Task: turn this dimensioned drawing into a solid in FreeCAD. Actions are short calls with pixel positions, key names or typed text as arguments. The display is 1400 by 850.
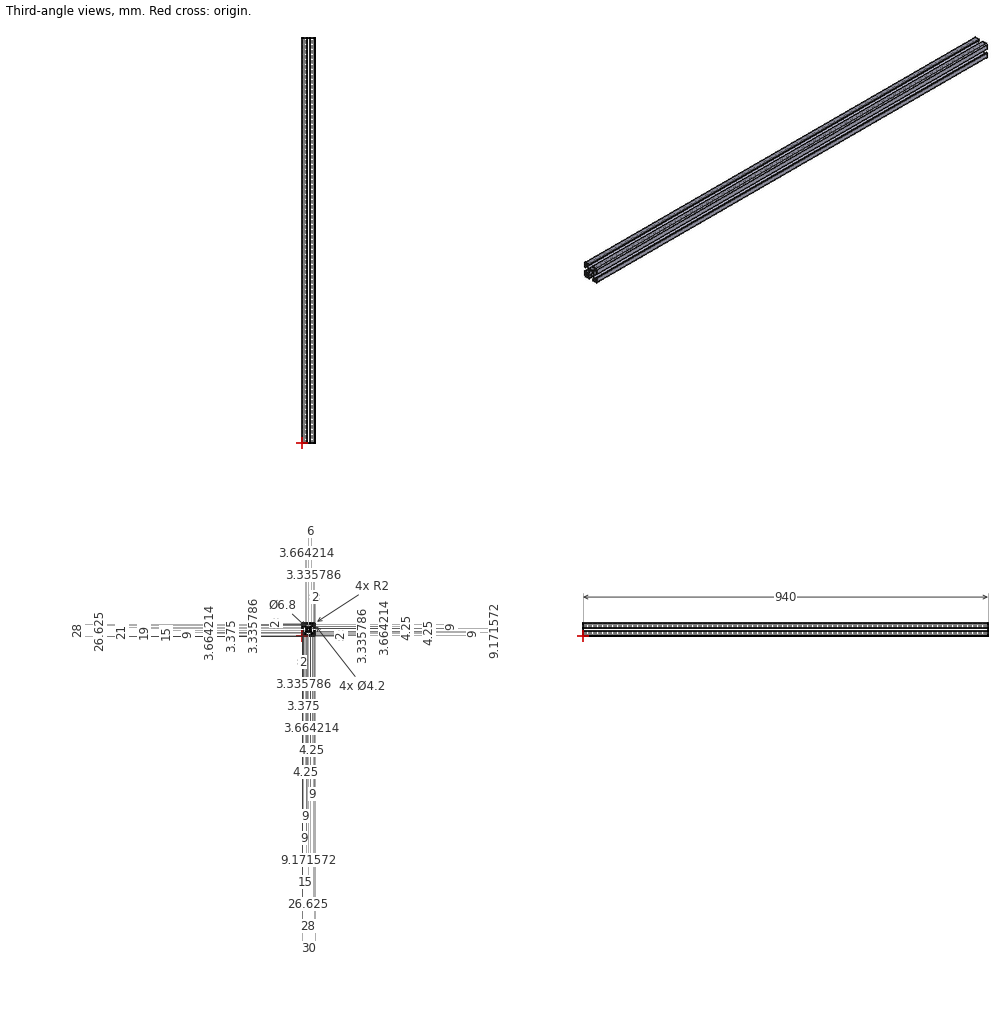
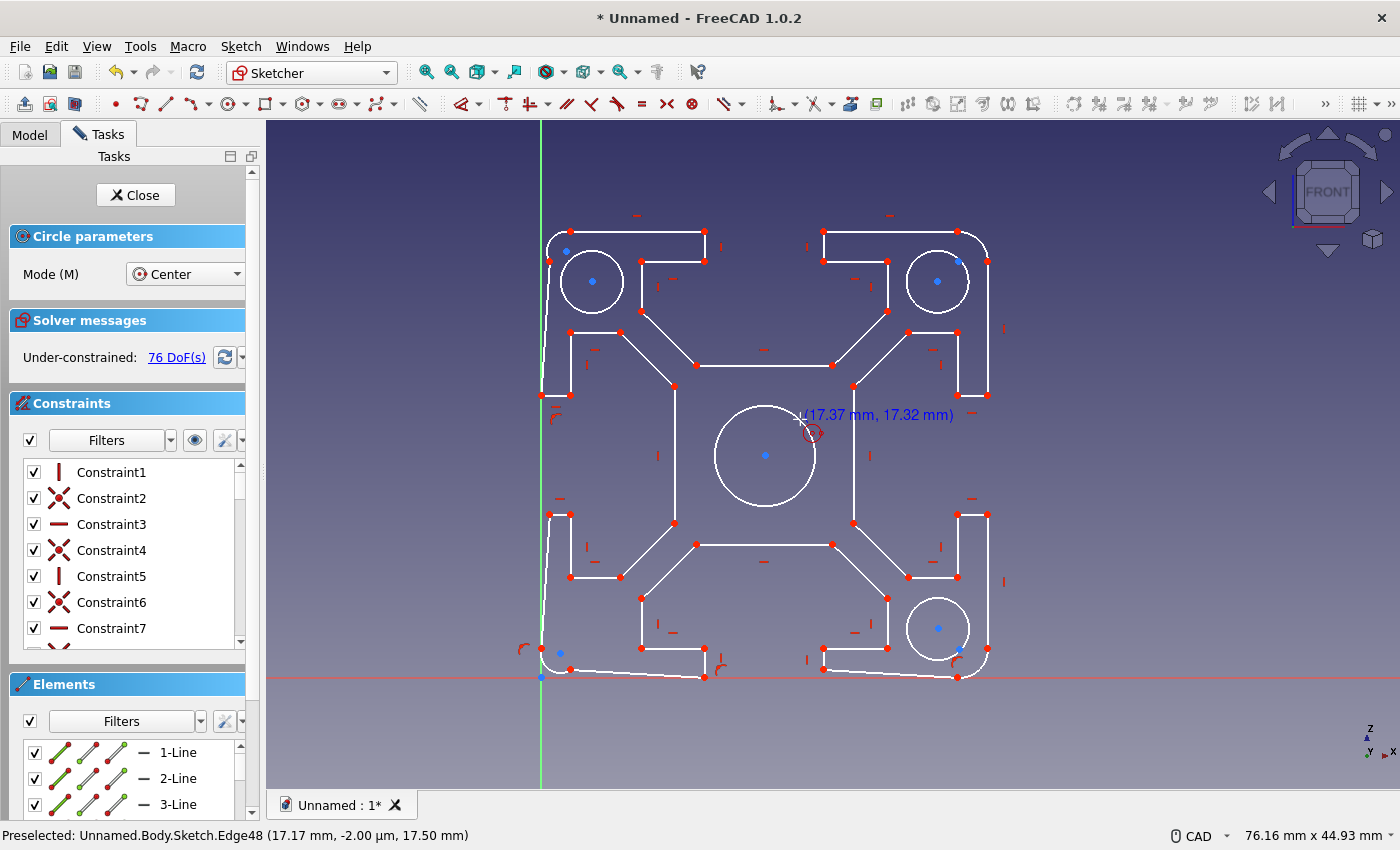
click(592, 628)
click(614, 606)
key(Escape)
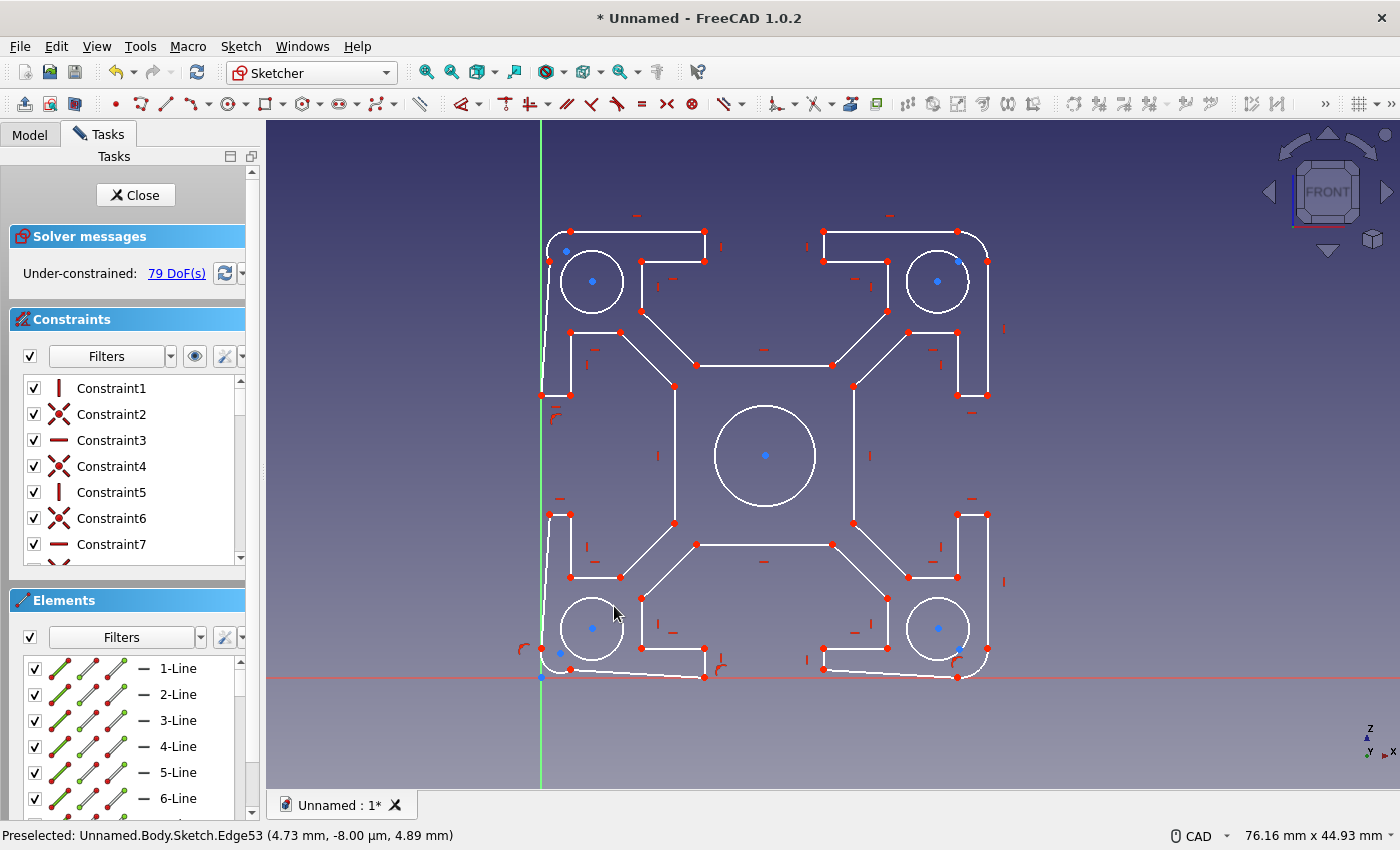
click(988, 302)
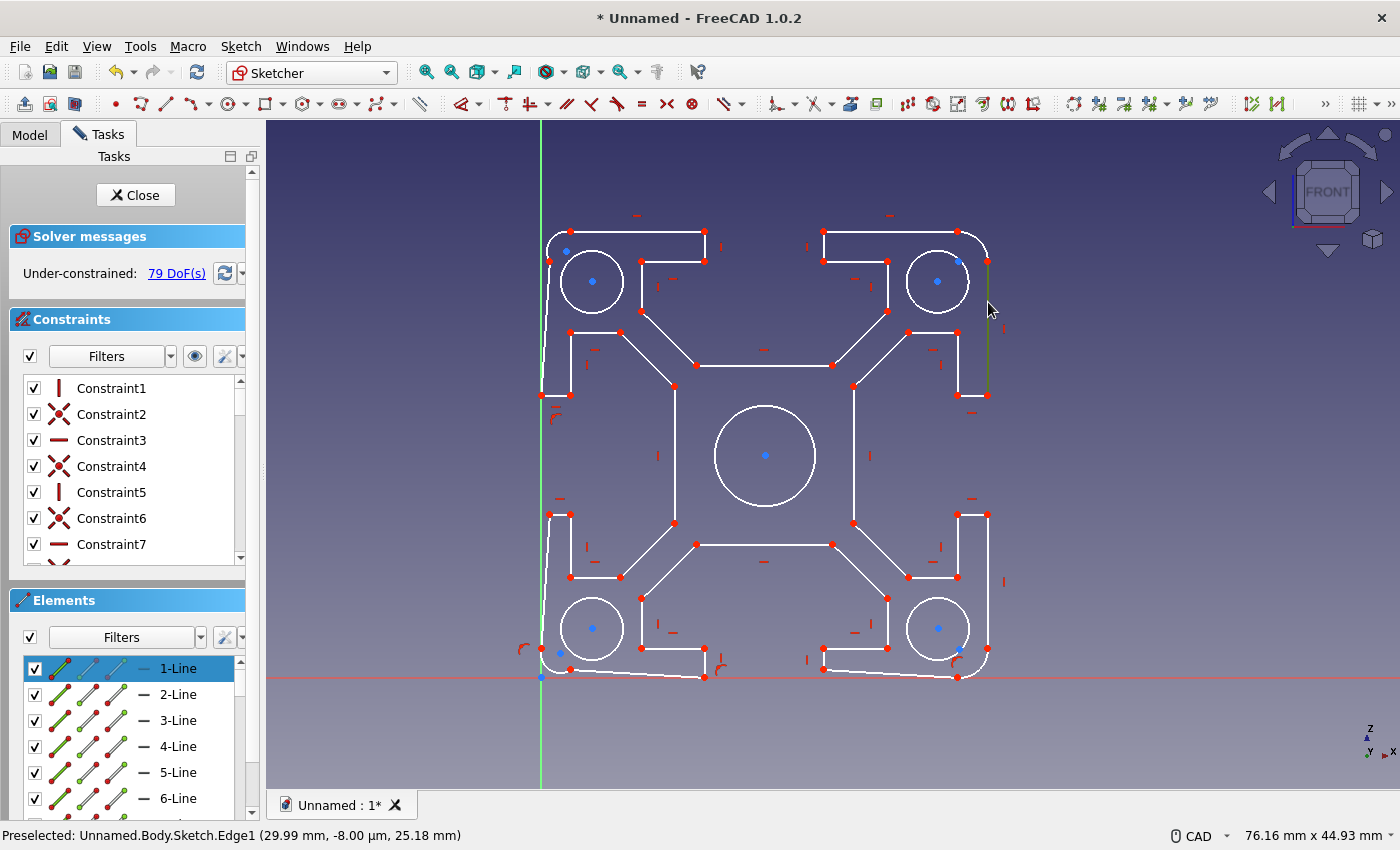
click(985, 248)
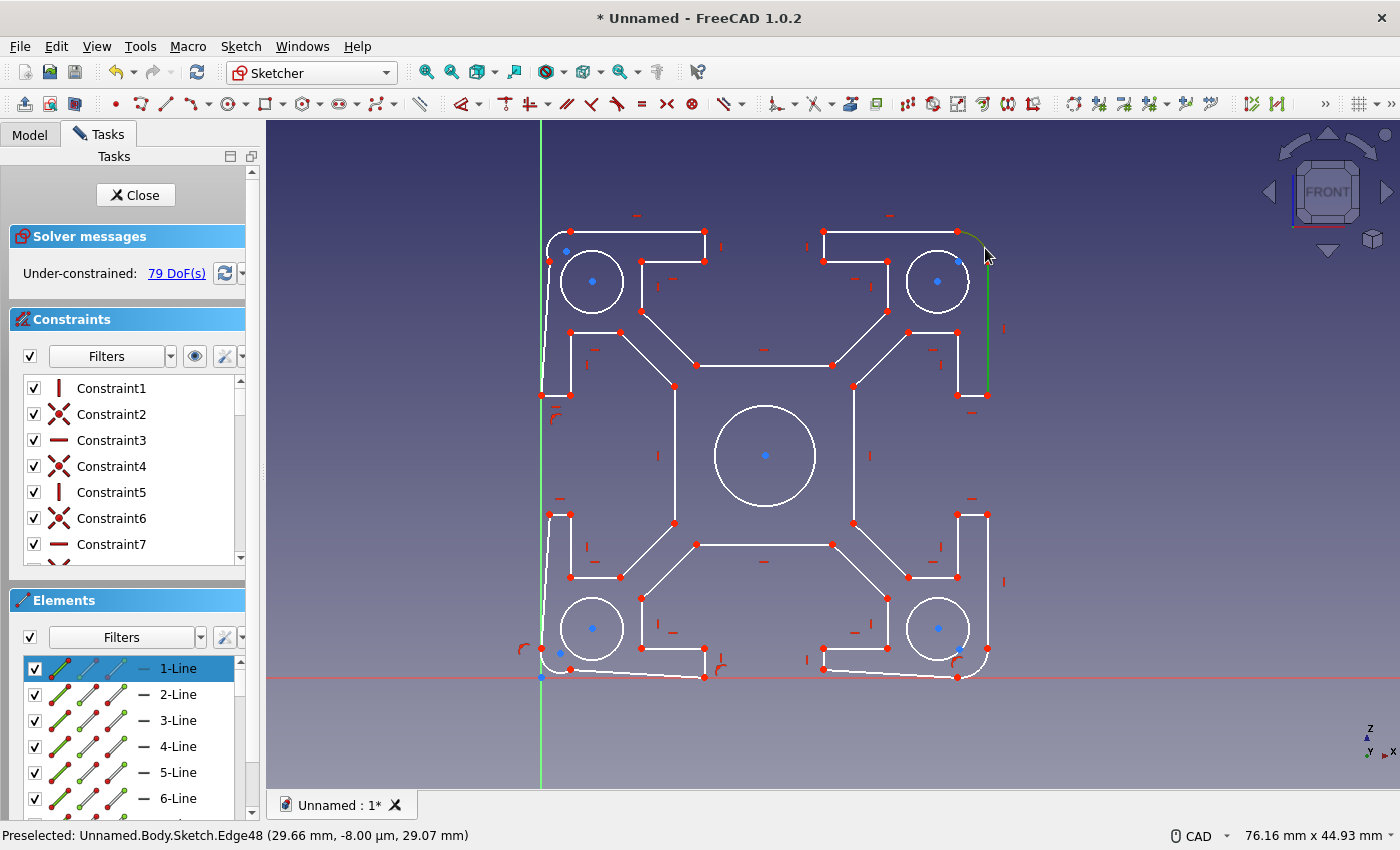
key(t)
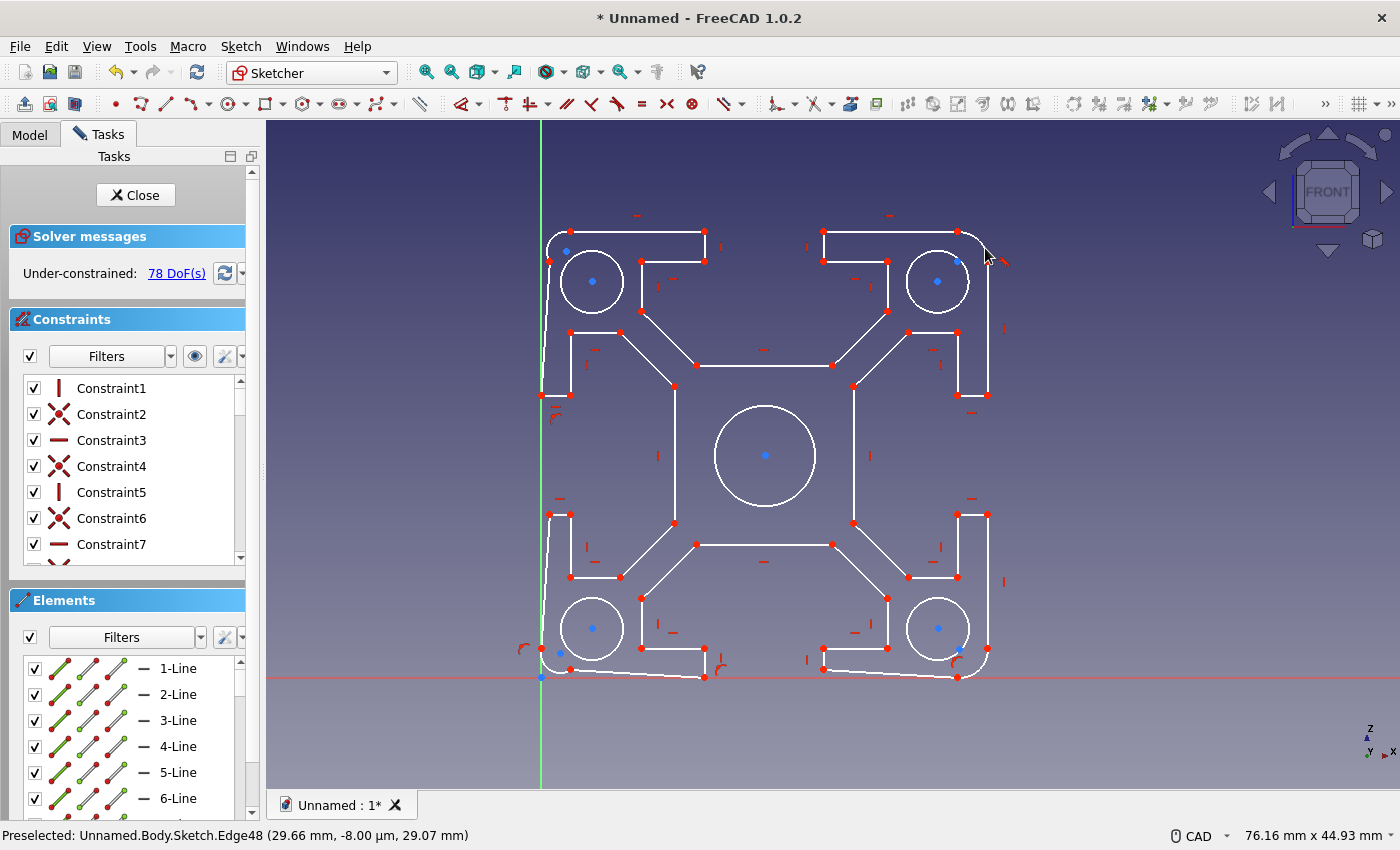
click(988, 555)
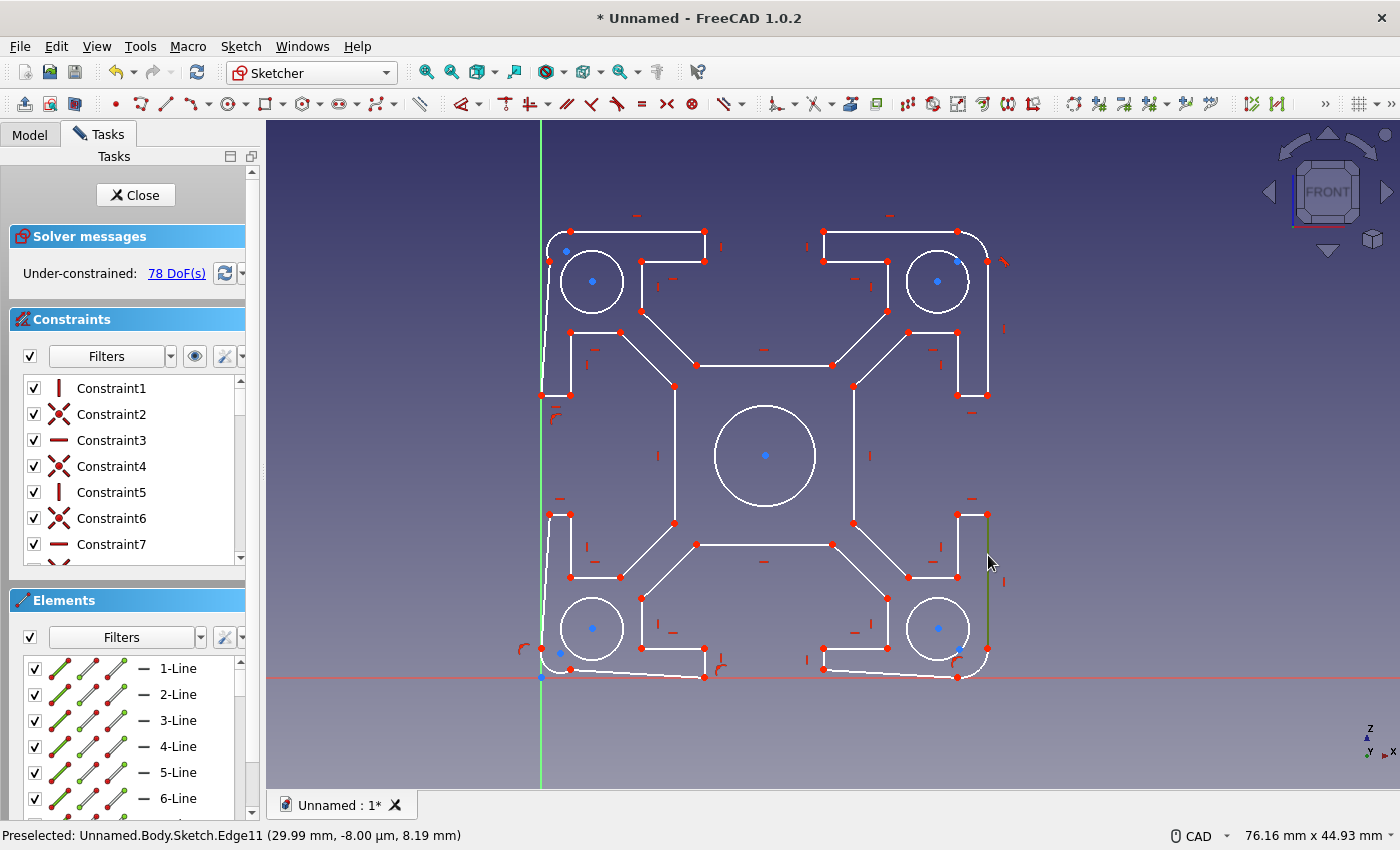
click(972, 675)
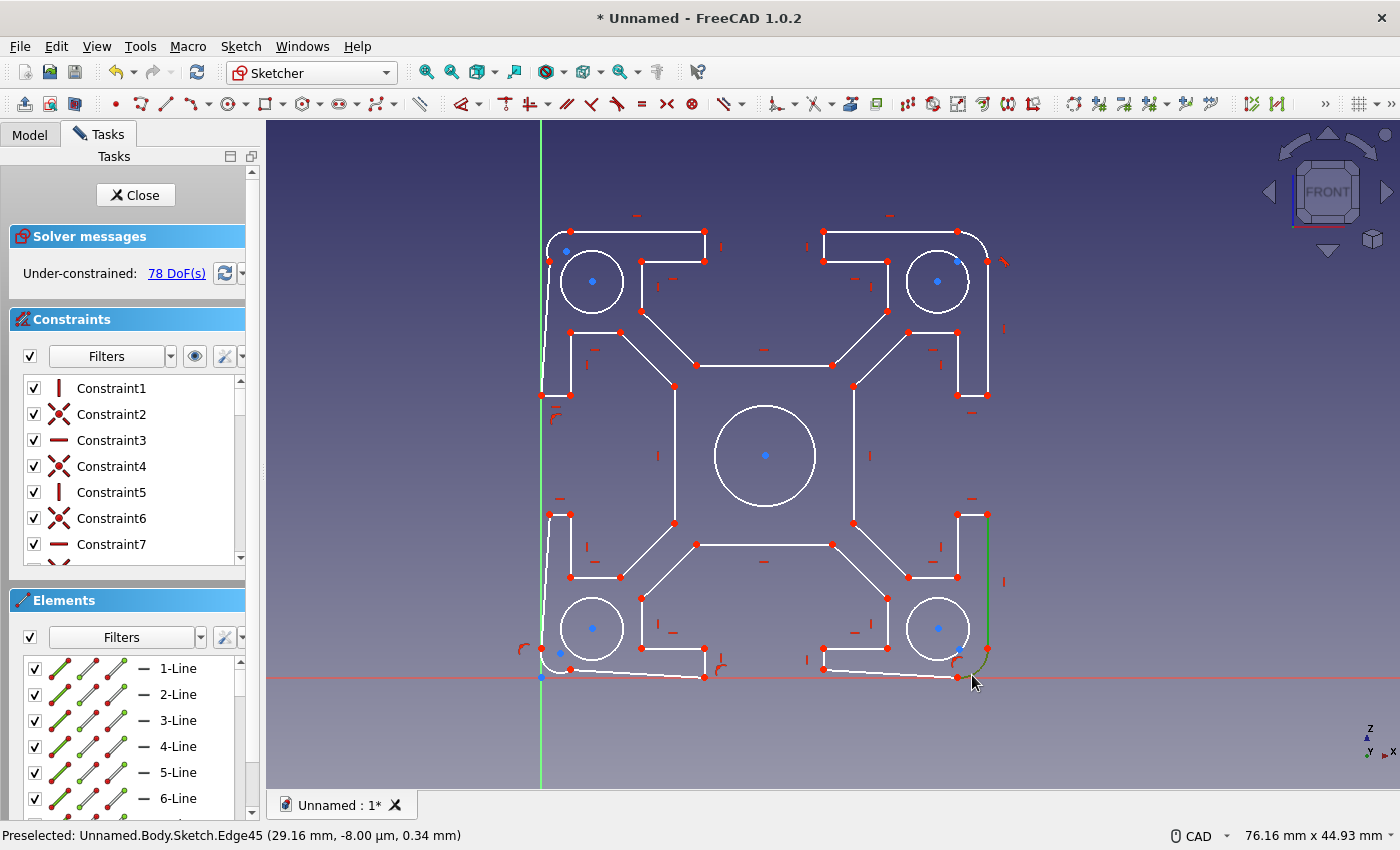
key(t)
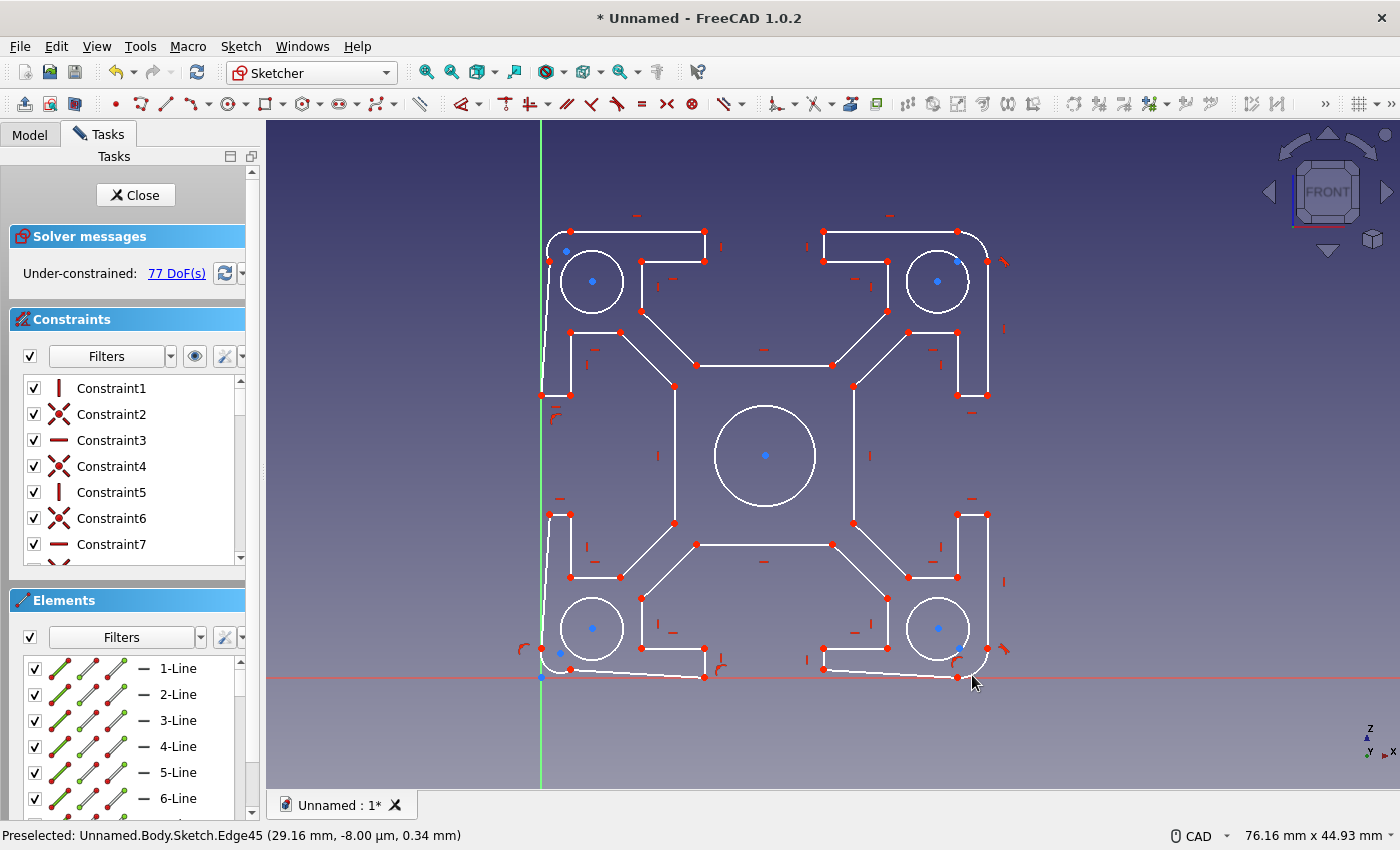
click(918, 676)